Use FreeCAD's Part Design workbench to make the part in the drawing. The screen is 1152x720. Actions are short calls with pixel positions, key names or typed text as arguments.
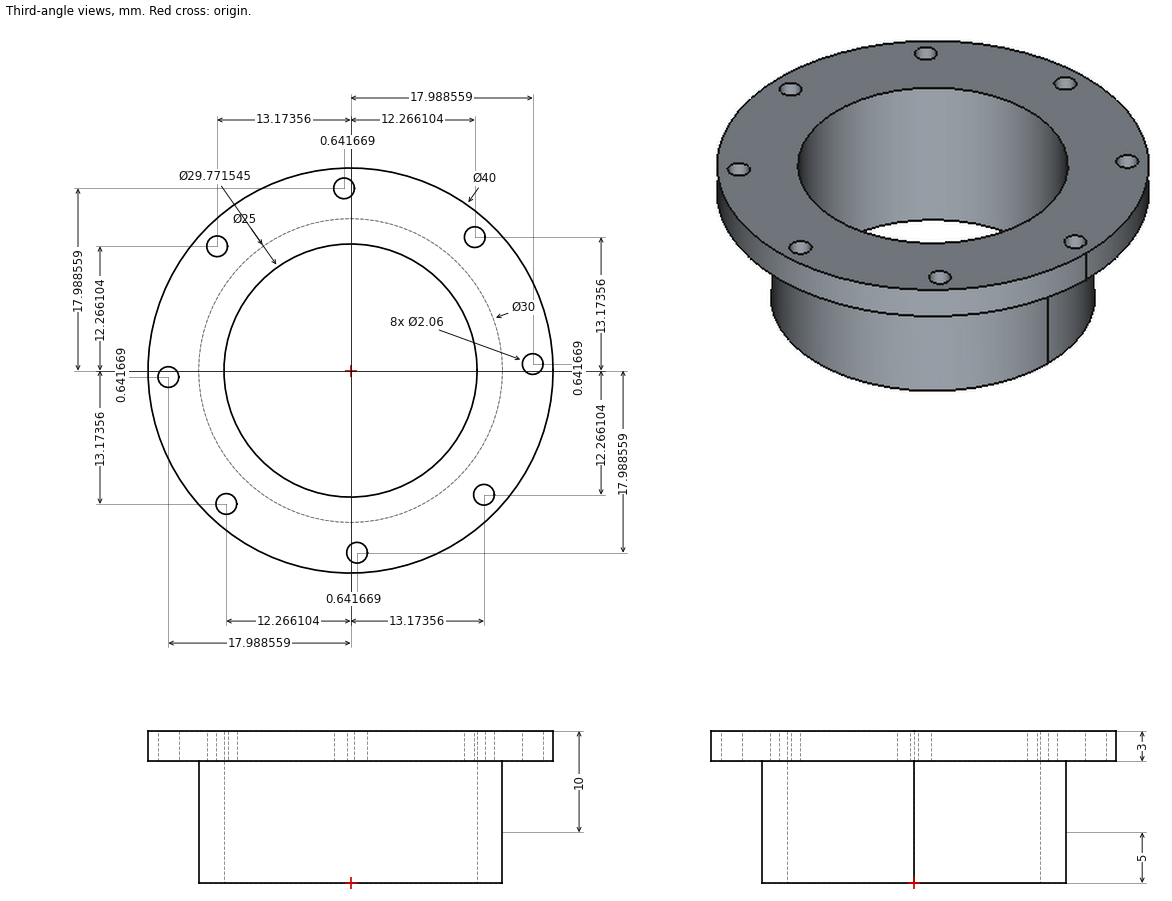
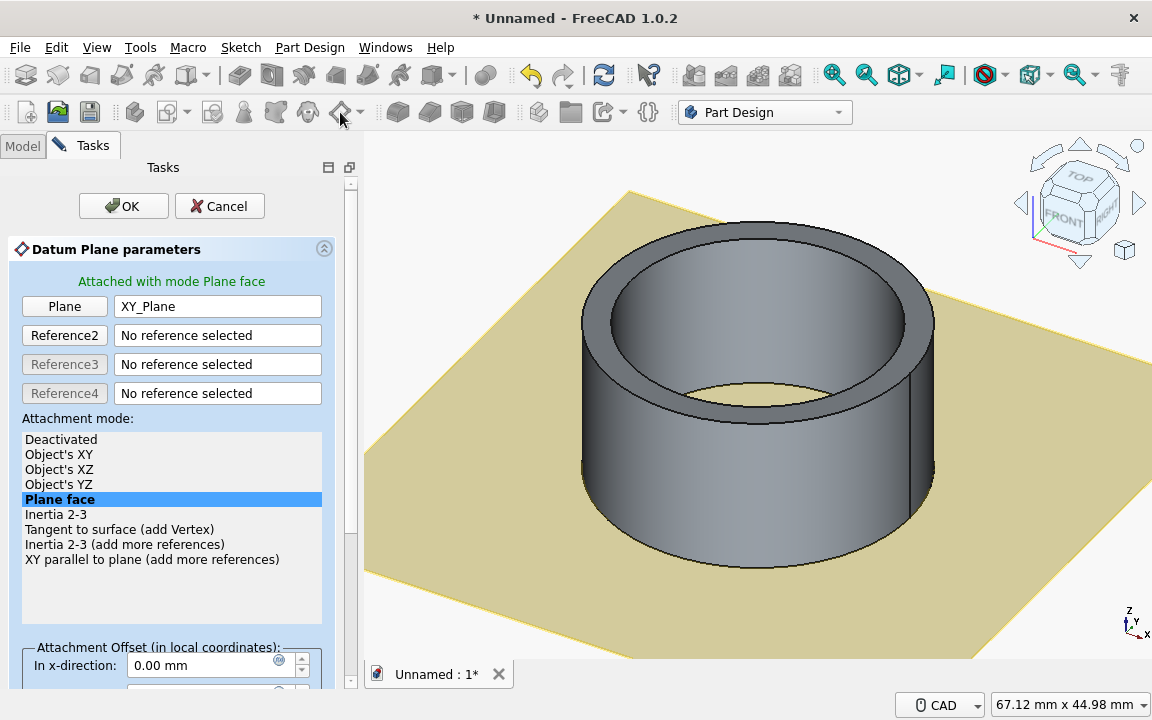
scroll(351, 432, down, 2)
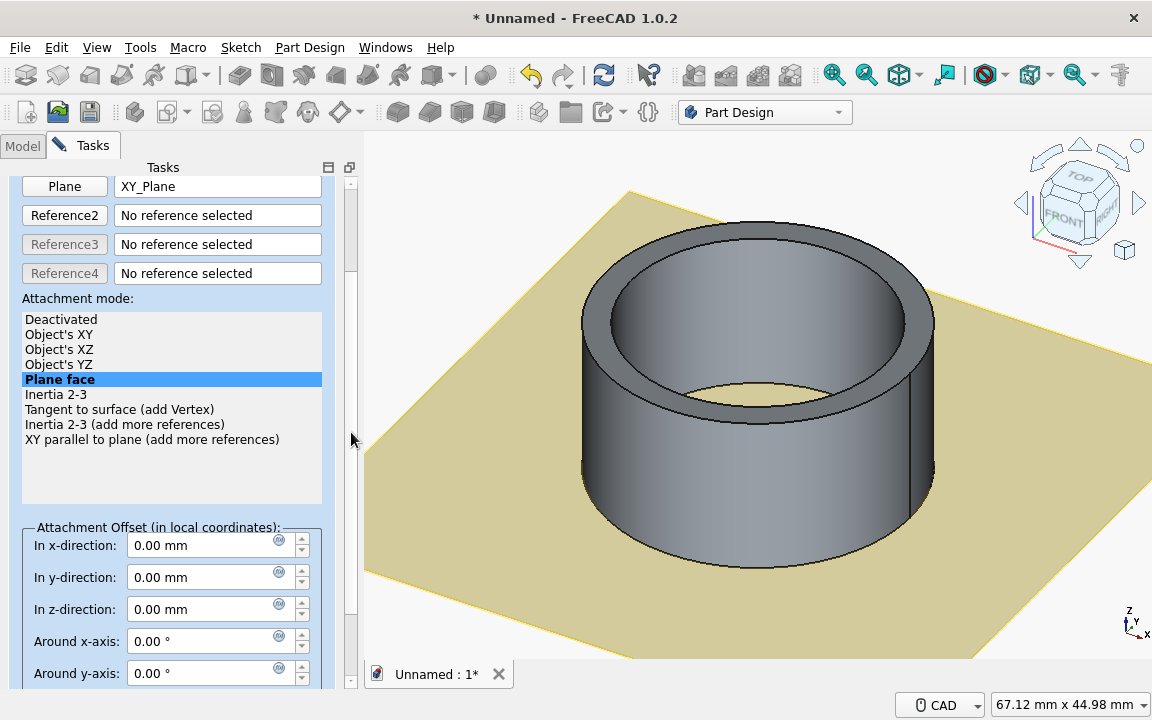
triple_click(210, 609)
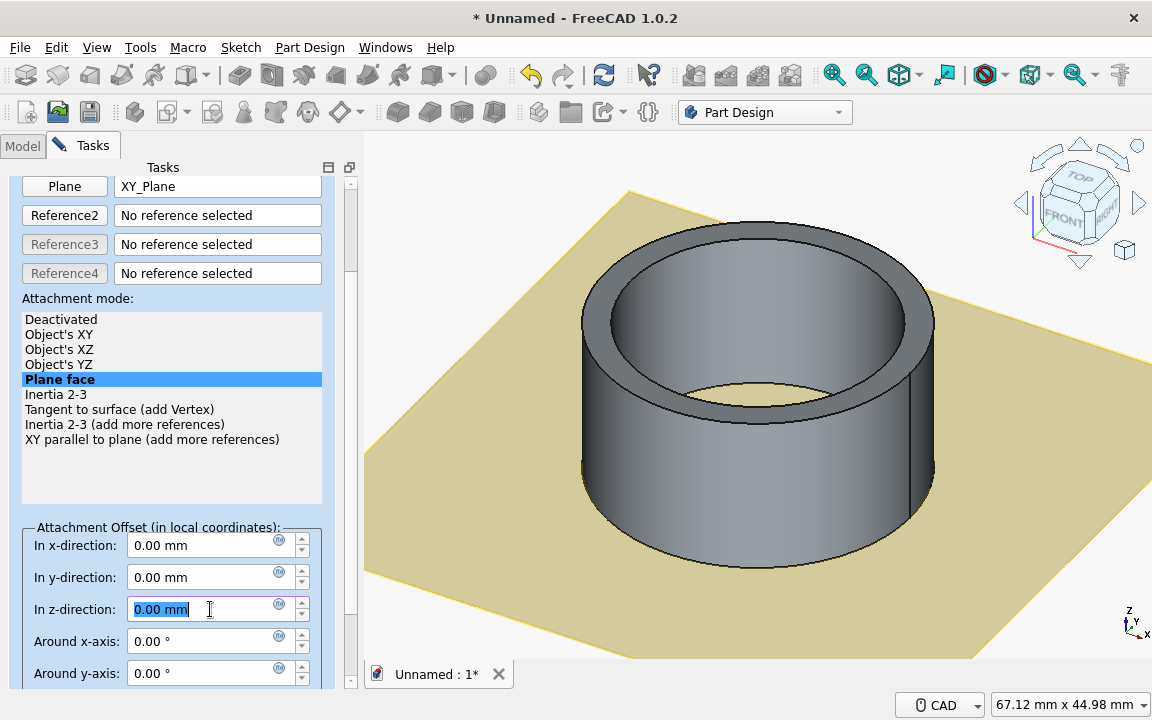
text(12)
key(Tab)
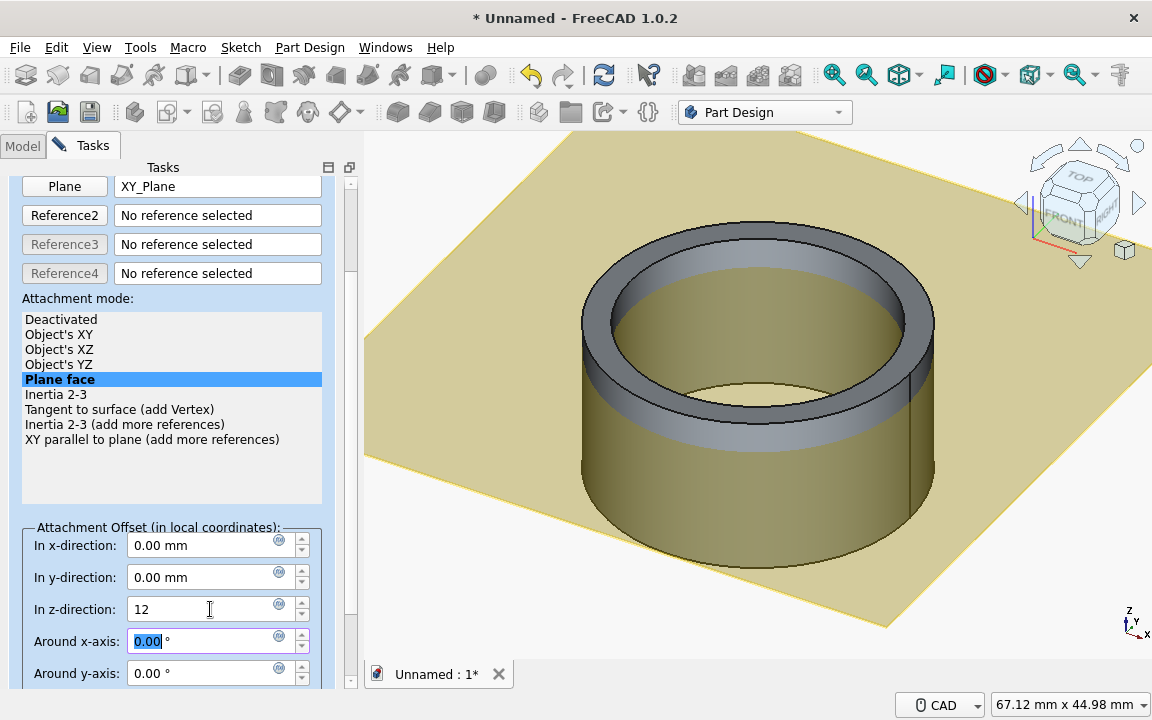
scroll(351, 432, up, 3)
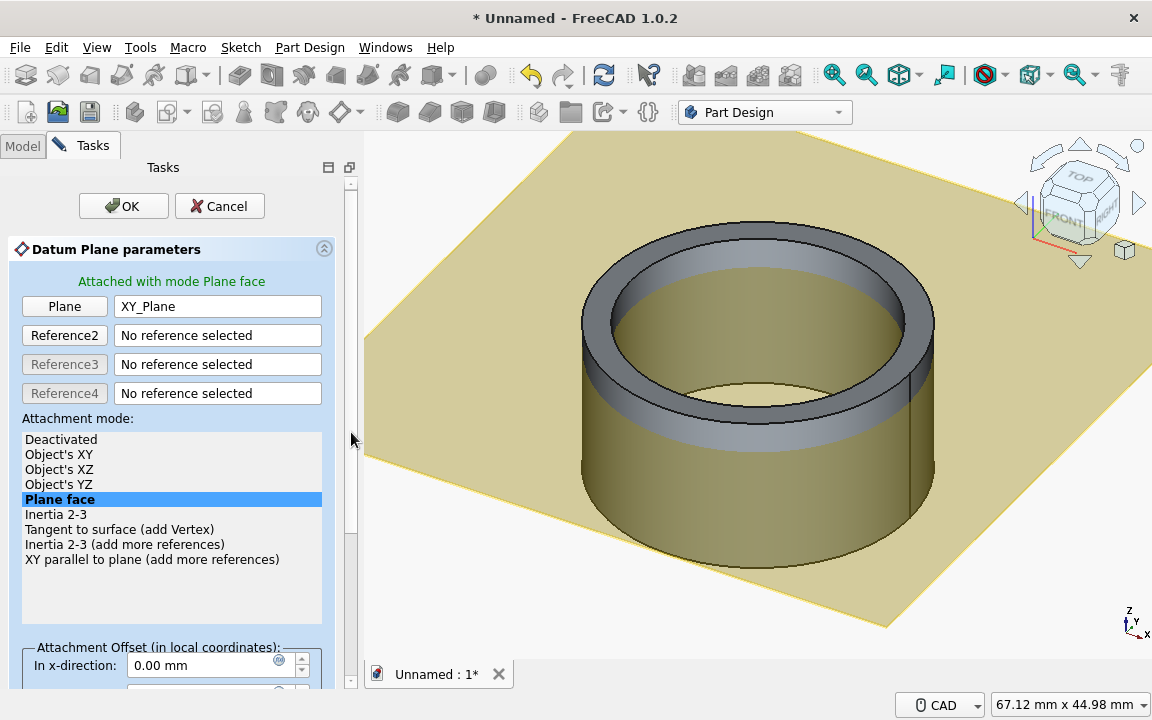
click(124, 206)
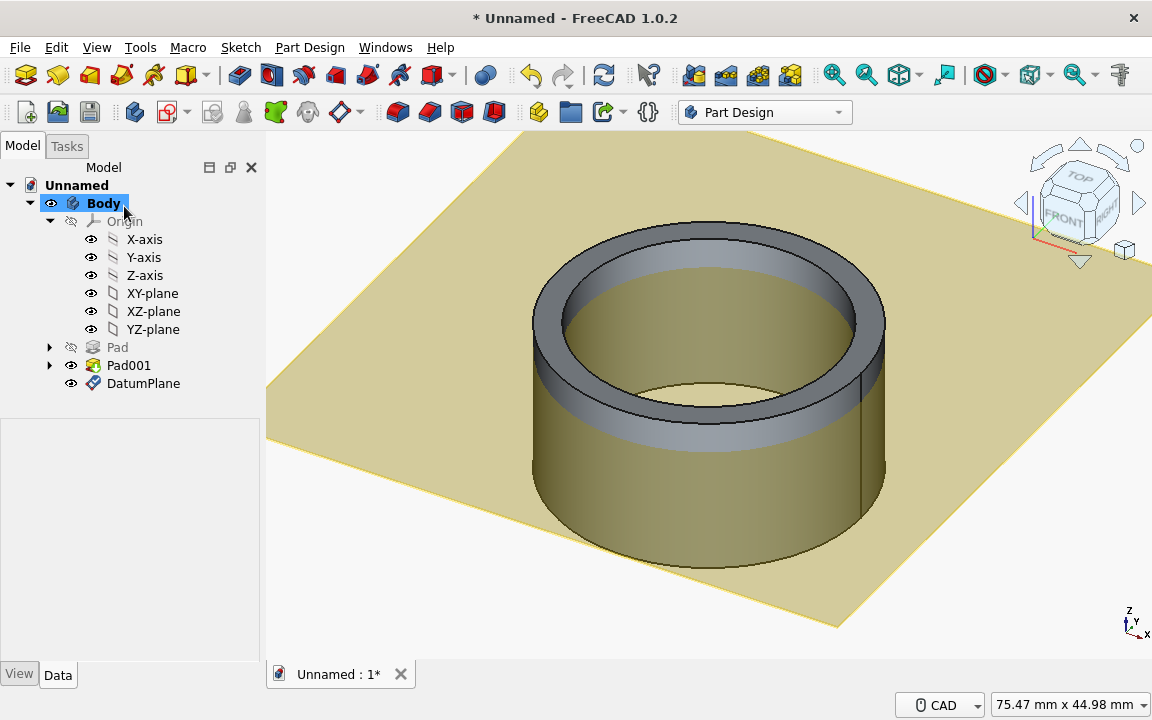
click(116, 383)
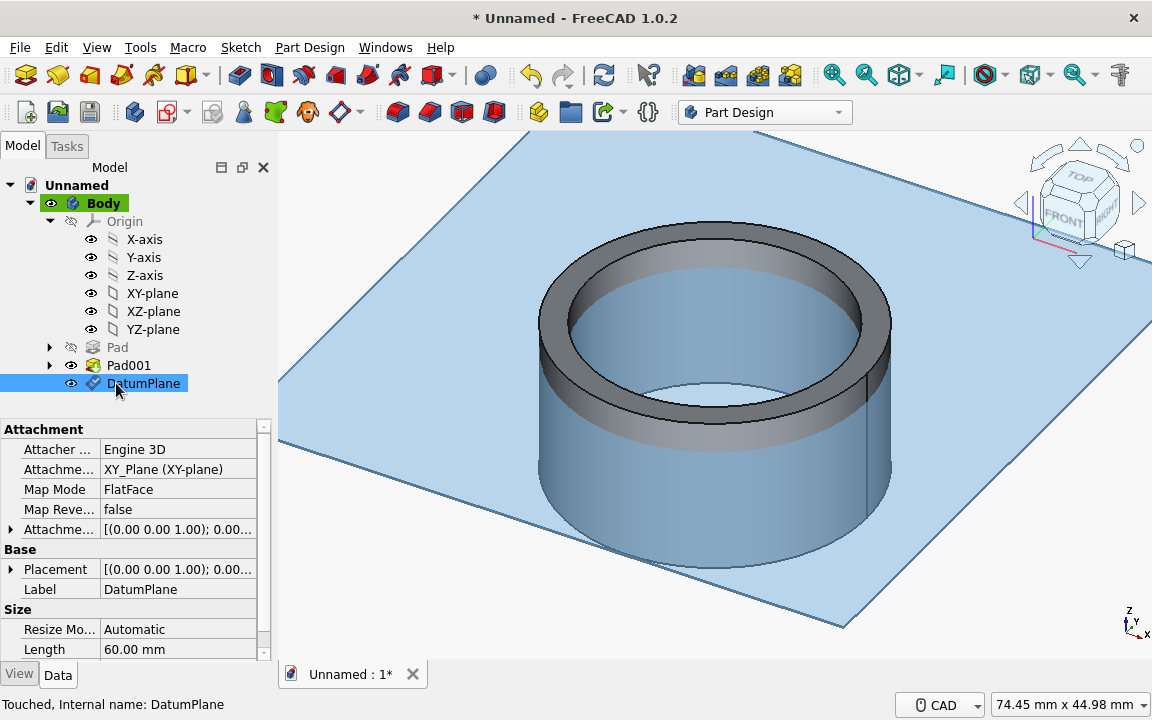
click(168, 112)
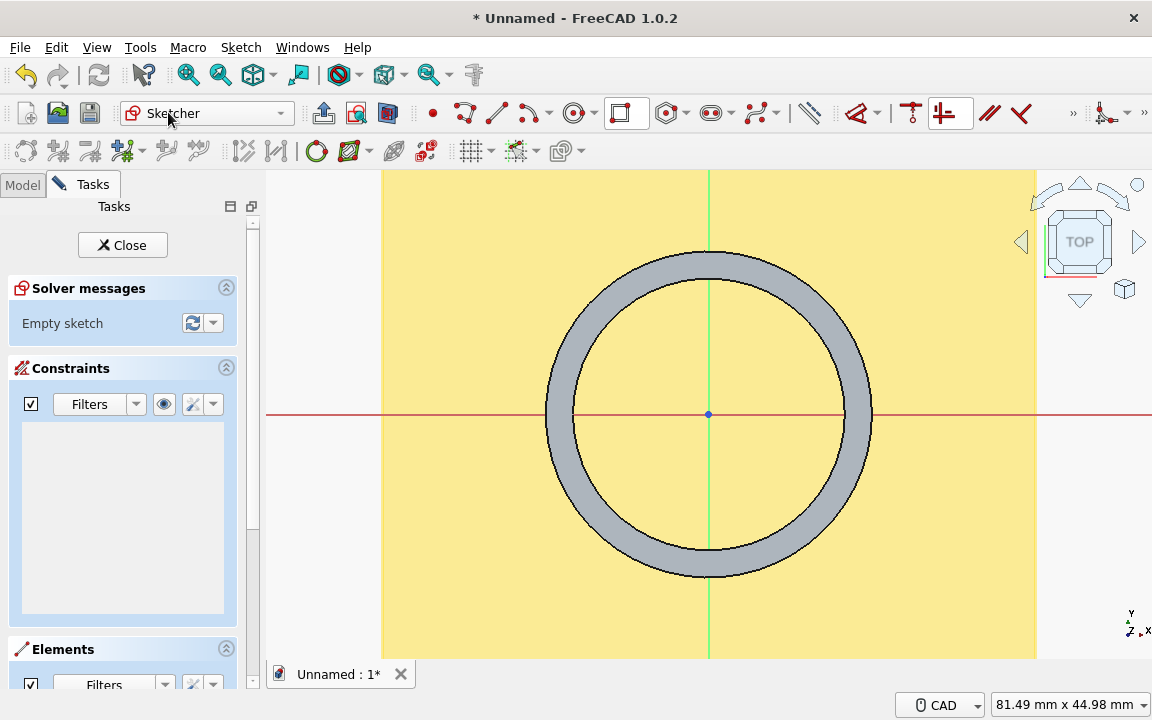
click(388, 114)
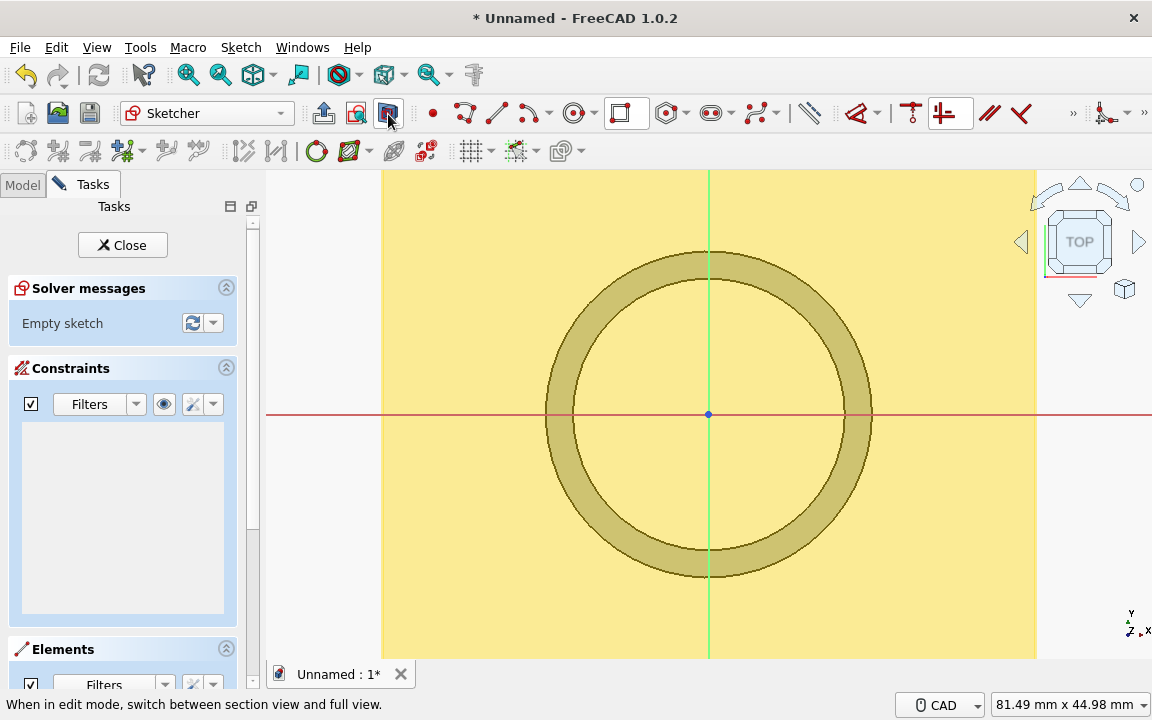
scroll(501, 414, down, 2)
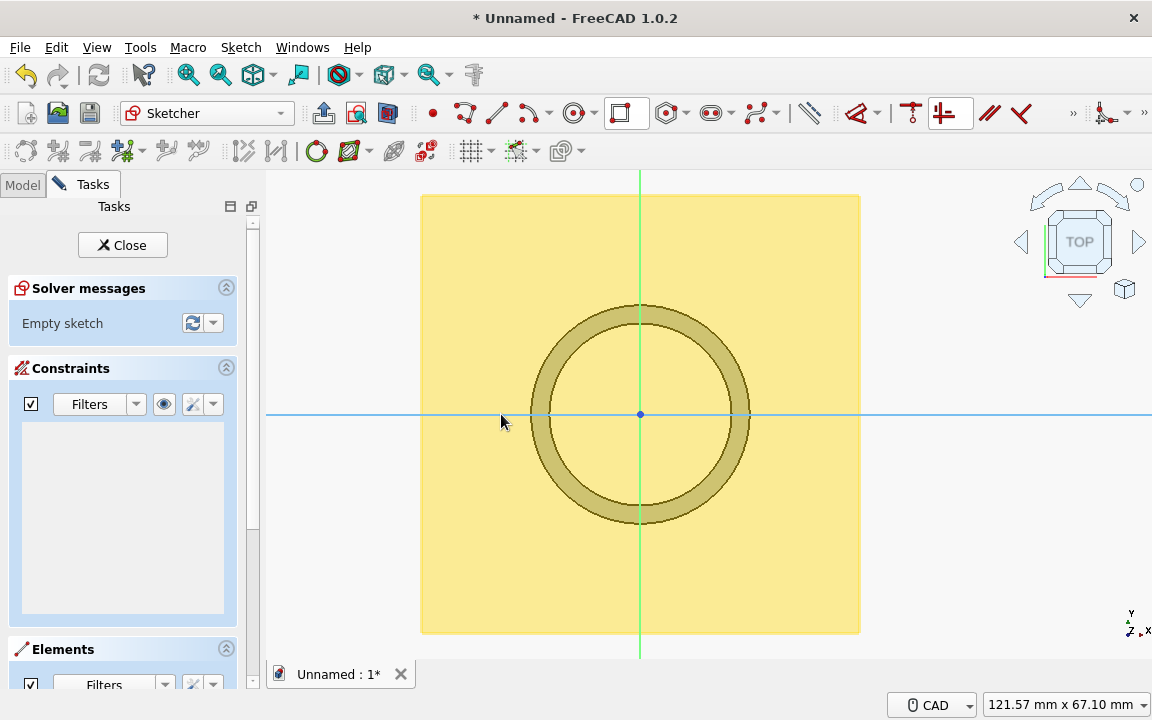
click(574, 114)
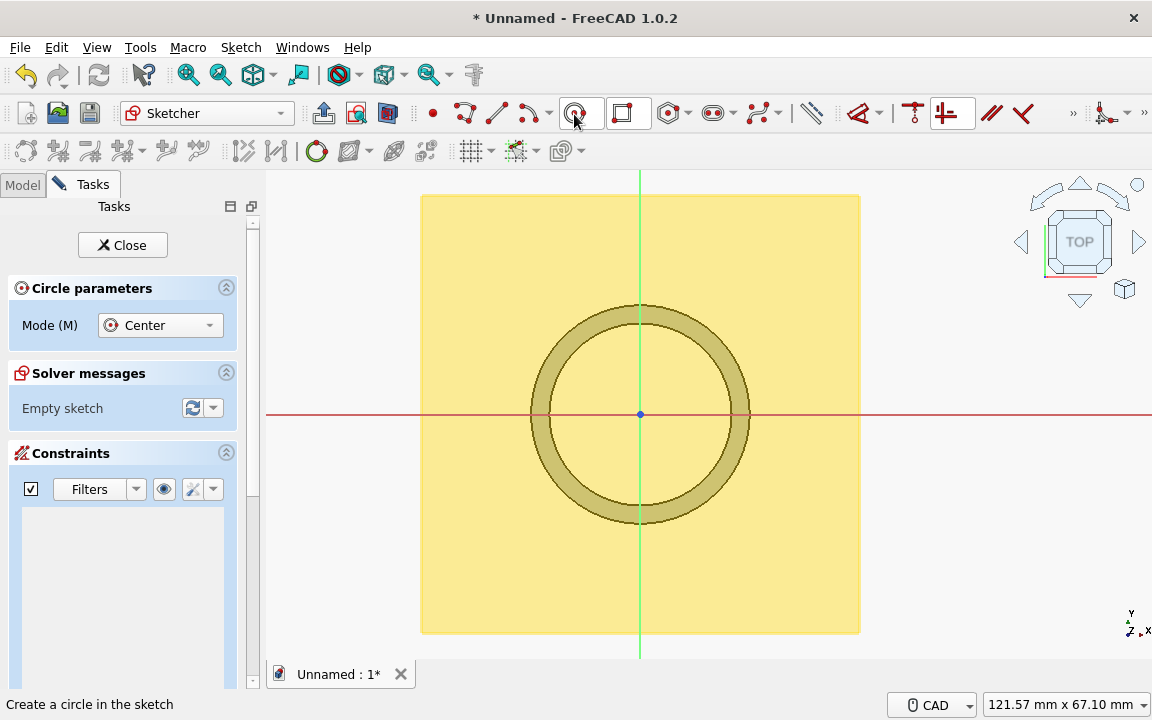
click(640, 414)
click(743, 311)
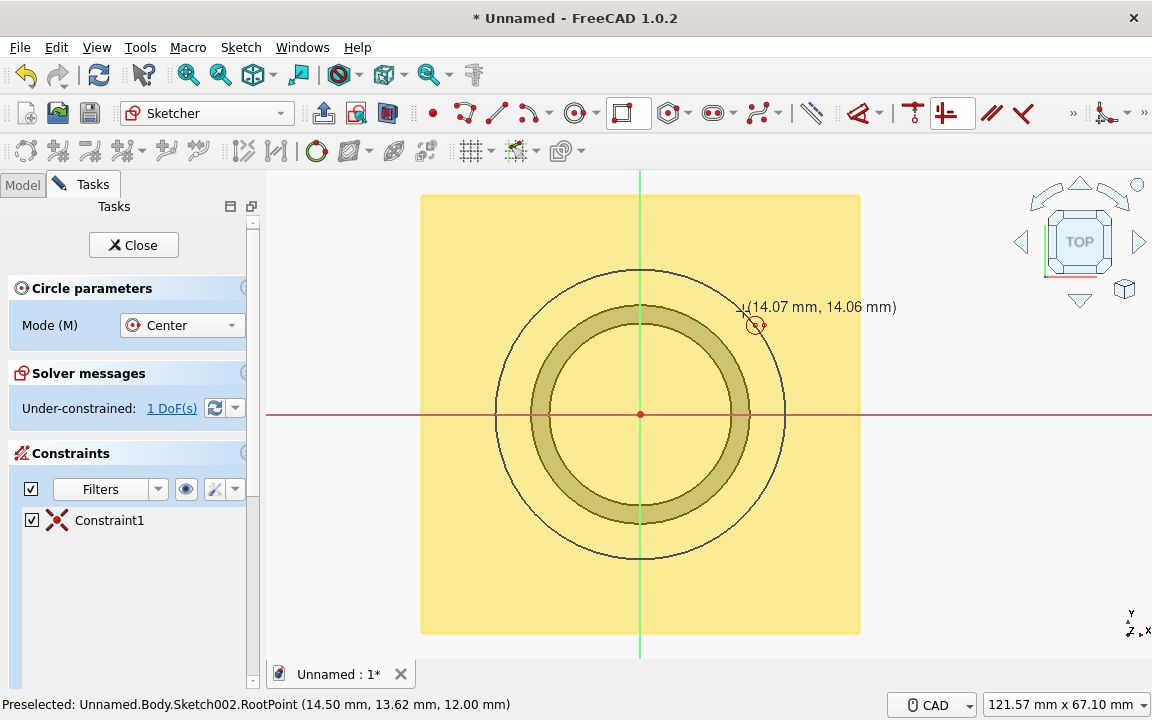
click(640, 414)
click(717, 338)
key(Escape)